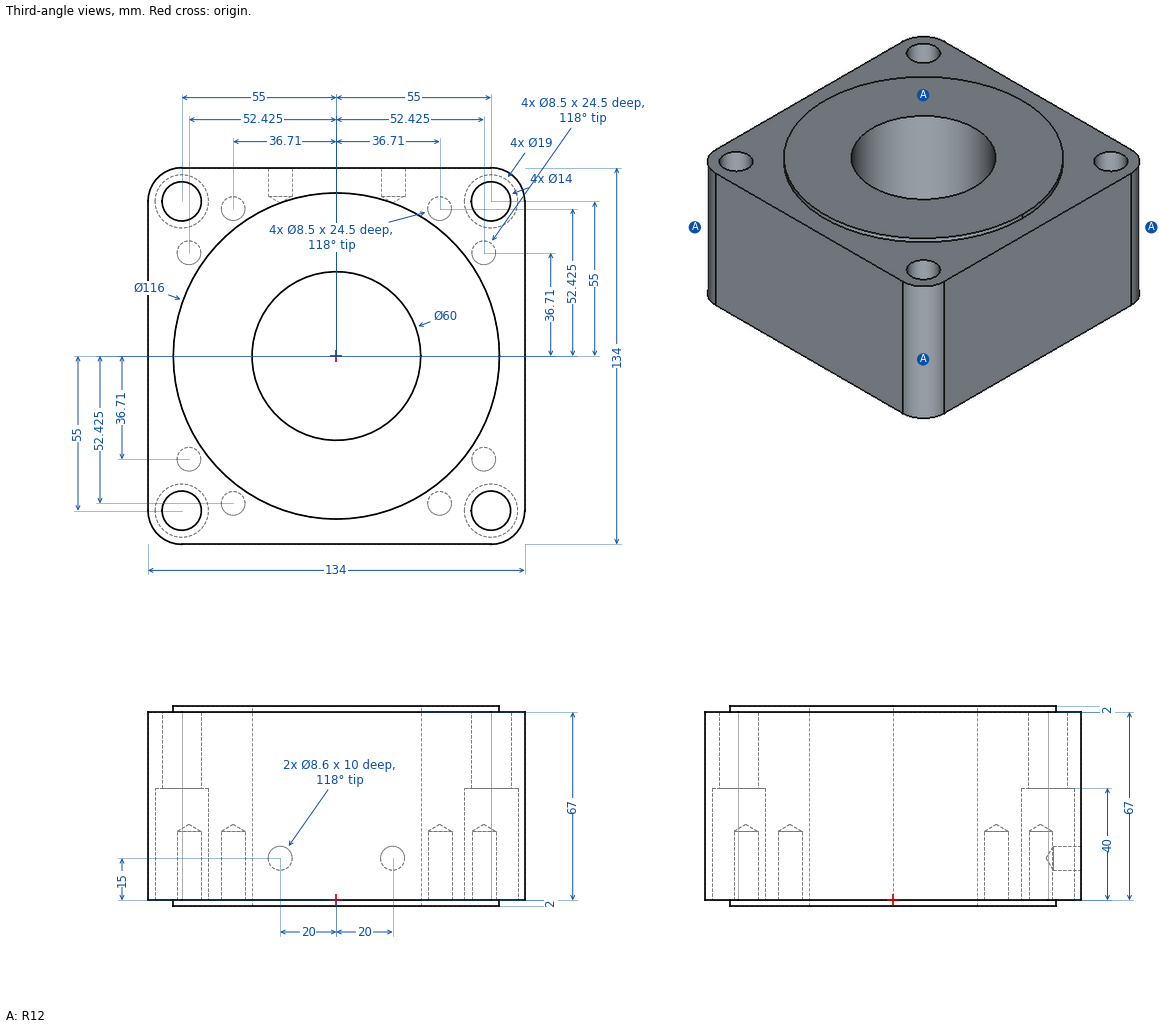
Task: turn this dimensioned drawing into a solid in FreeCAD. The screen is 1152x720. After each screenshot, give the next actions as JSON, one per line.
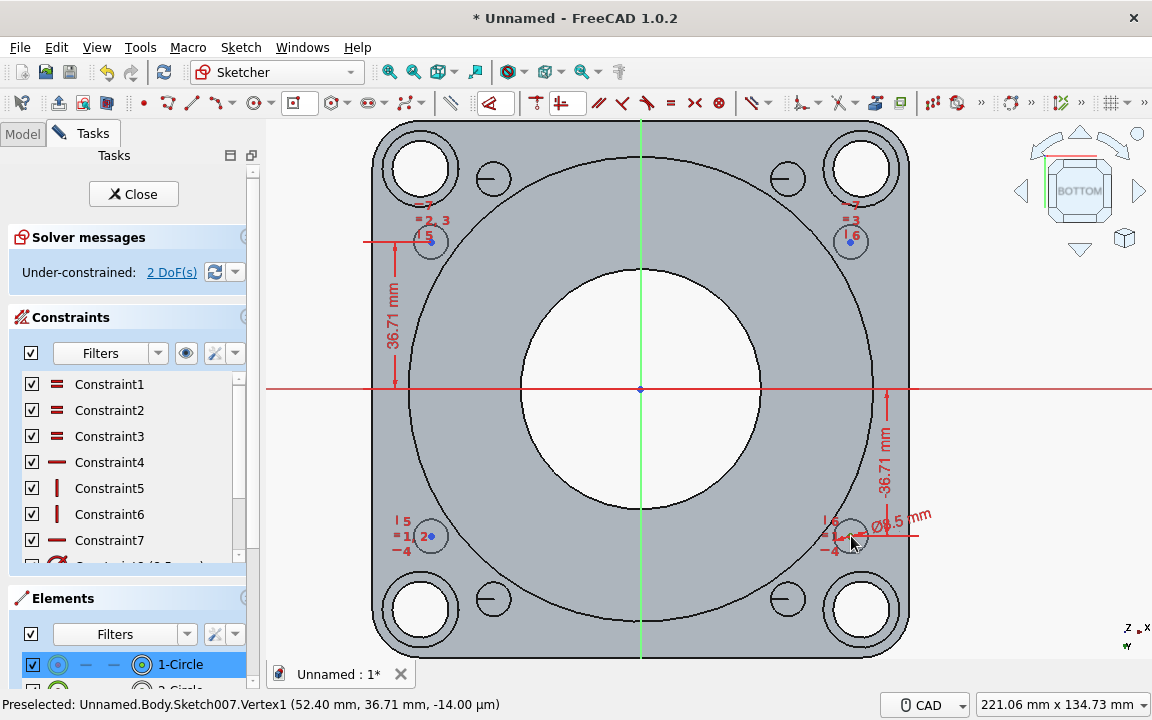
{"action": "left_click", "coordinate": [508, 104]}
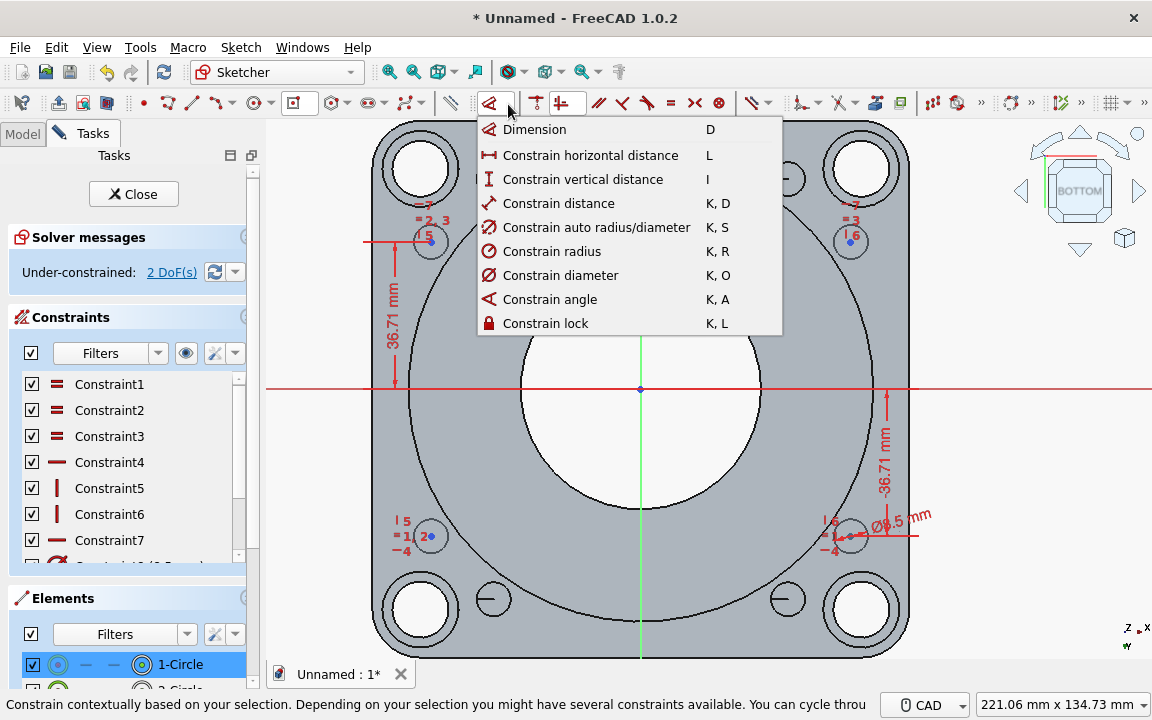
{"action": "left_click", "coordinate": [630, 155]}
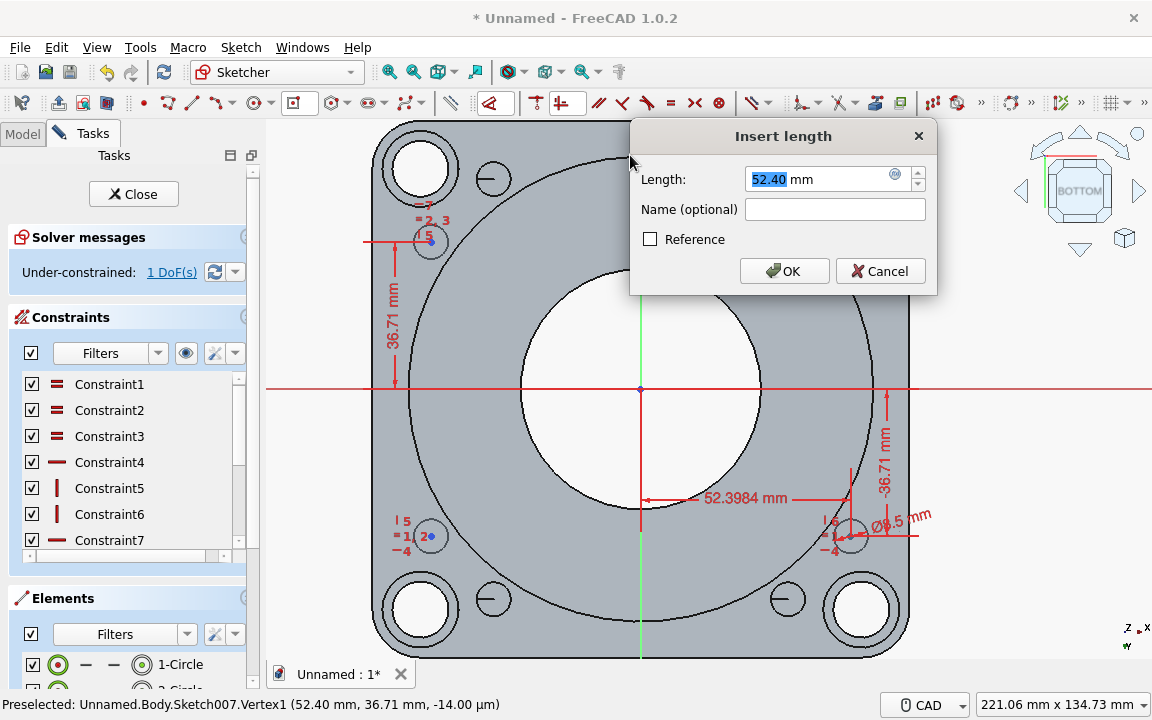
{"action": "type", "text": "52.425"}
{"action": "key", "text": "Return"}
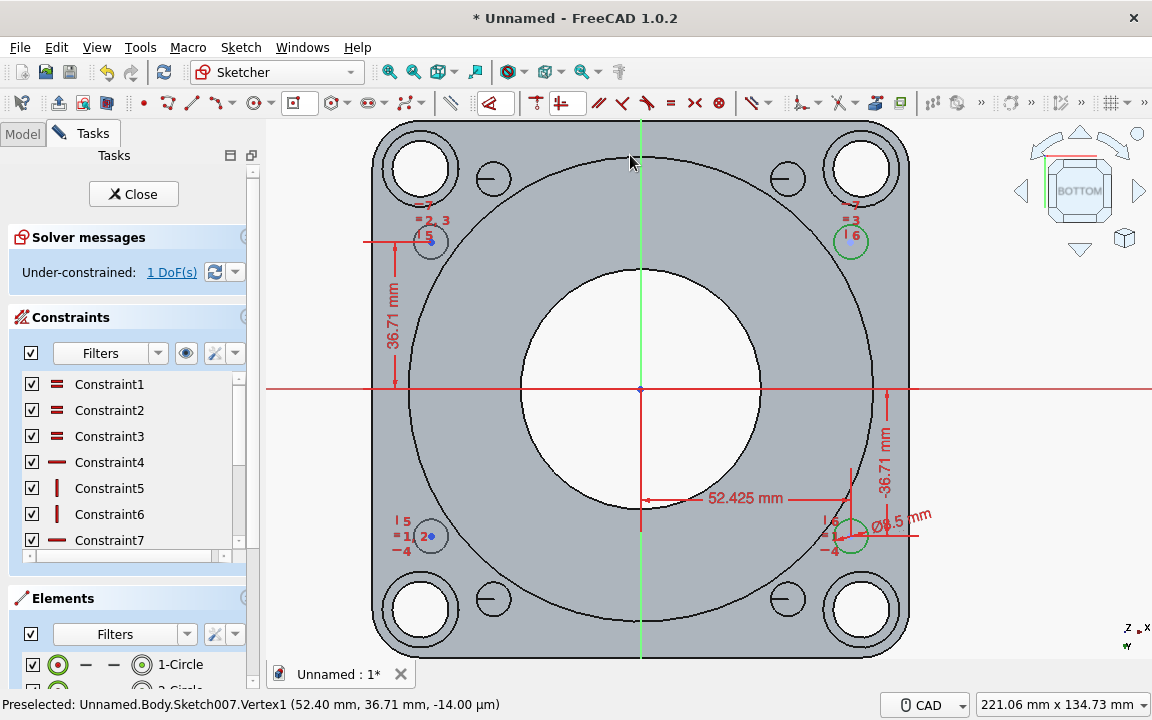
{"action": "left_click", "coordinate": [431, 536]}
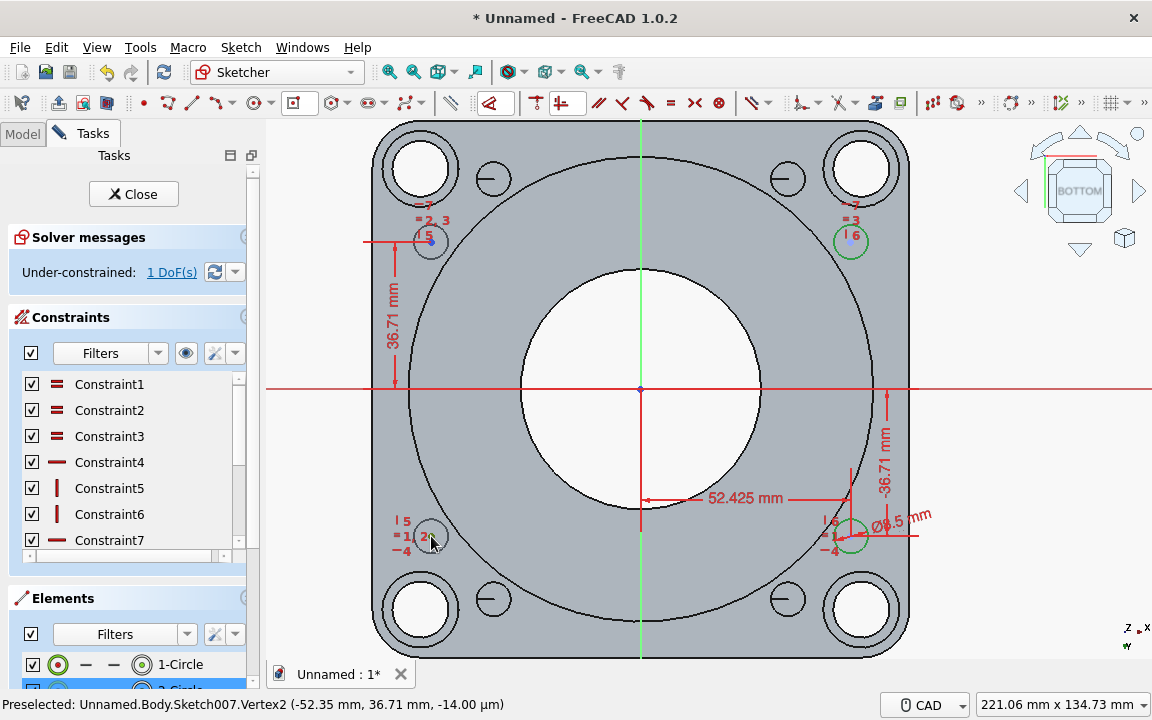
{"action": "left_click", "coordinate": [508, 104]}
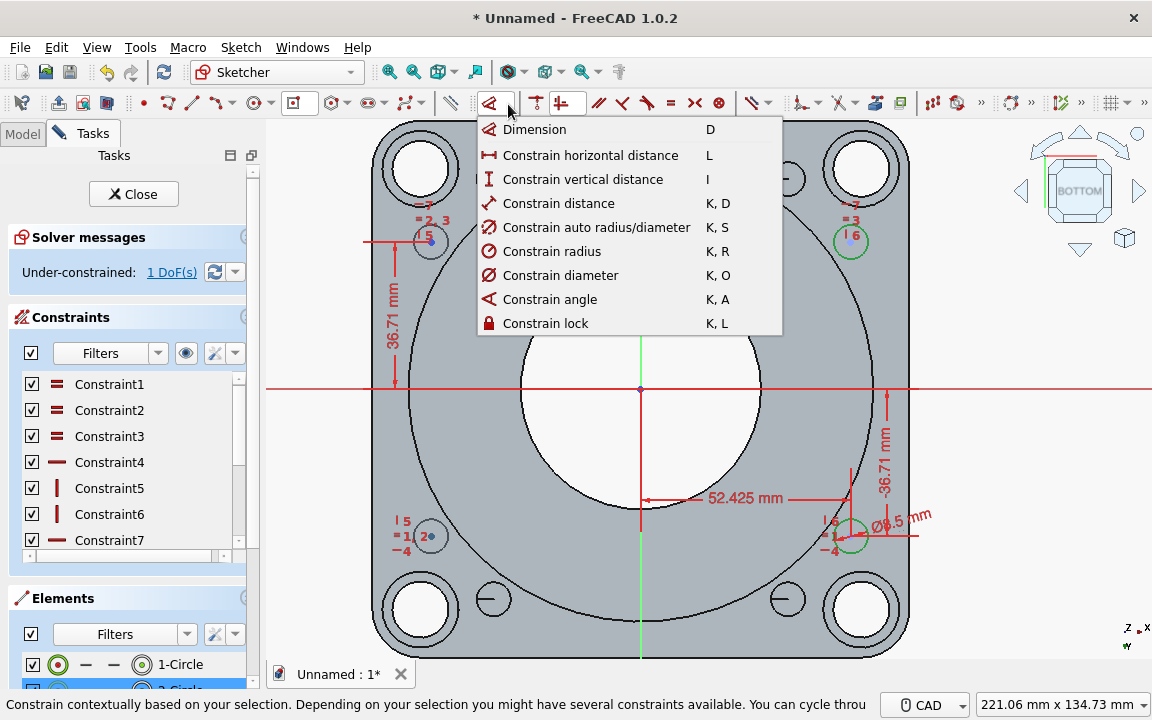
{"action": "left_click", "coordinate": [630, 155]}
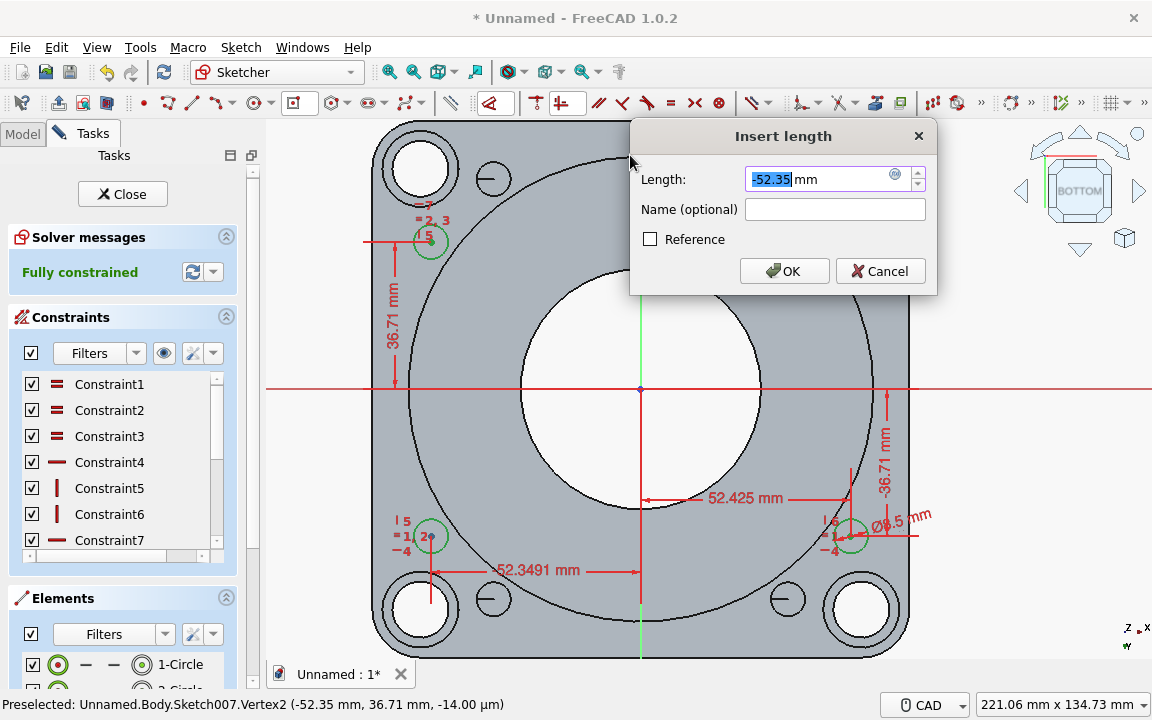
{"action": "type", "text": "-52.425"}
{"action": "key", "text": "Return"}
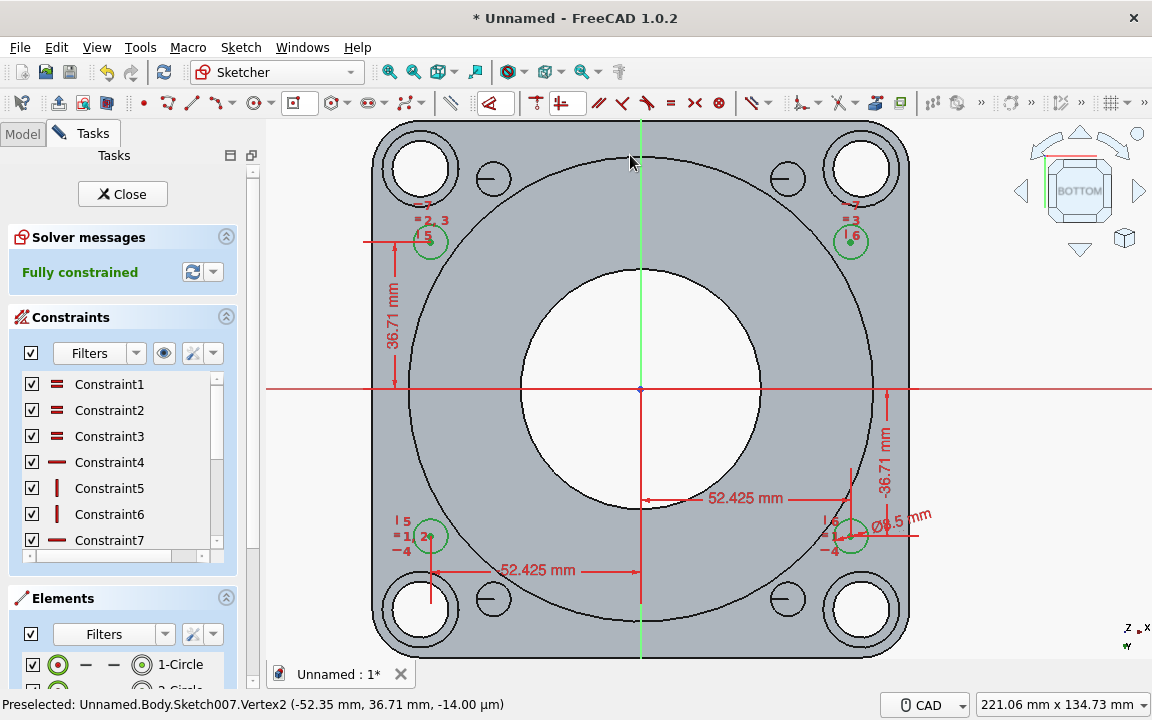
{"action": "left_click", "coordinate": [123, 194]}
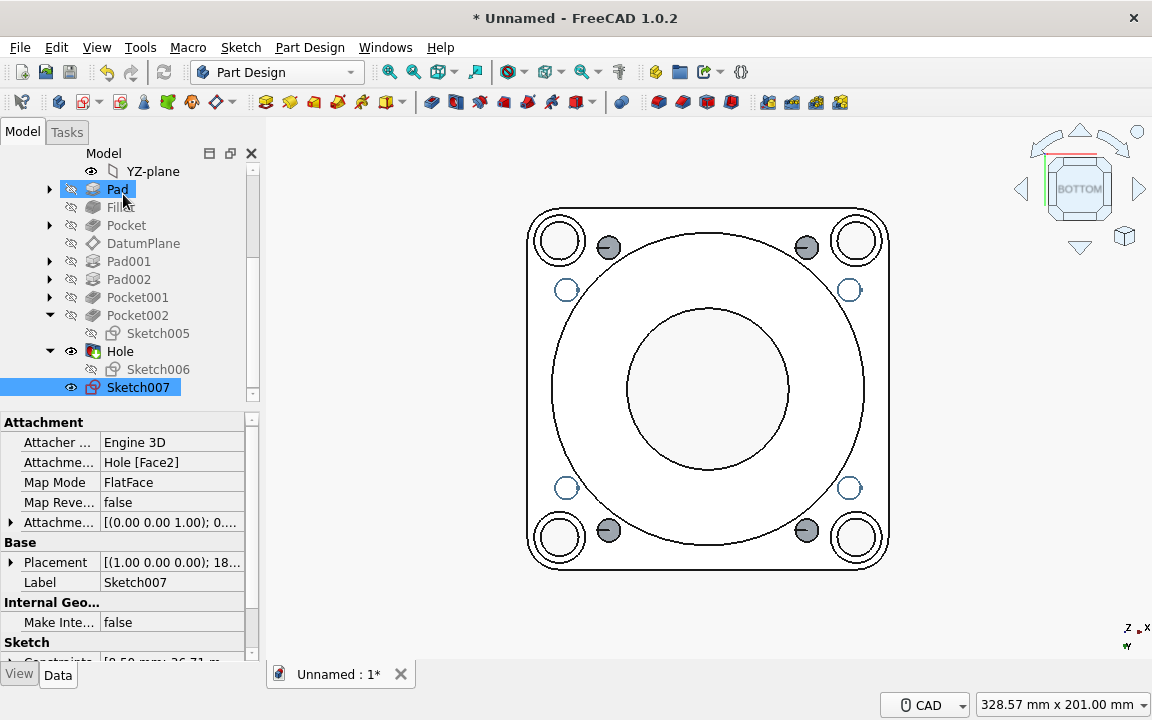
{"action": "left_click", "coordinate": [456, 102]}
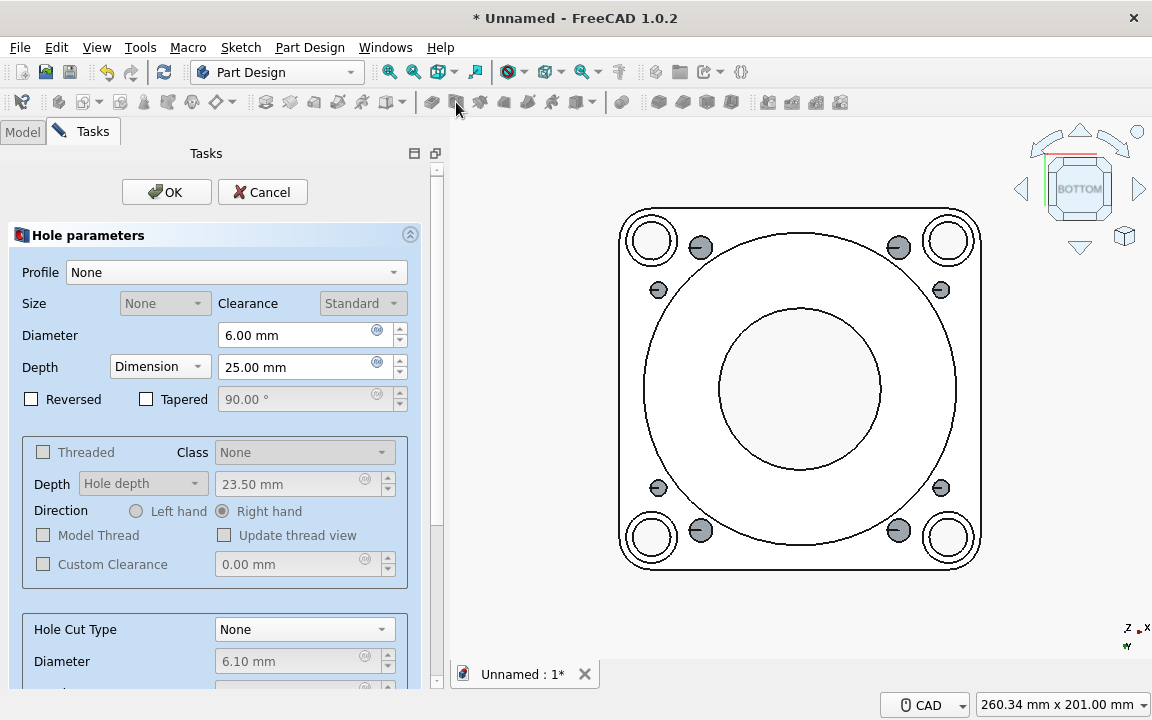
{"action": "triple_click", "coordinate": [305, 335]}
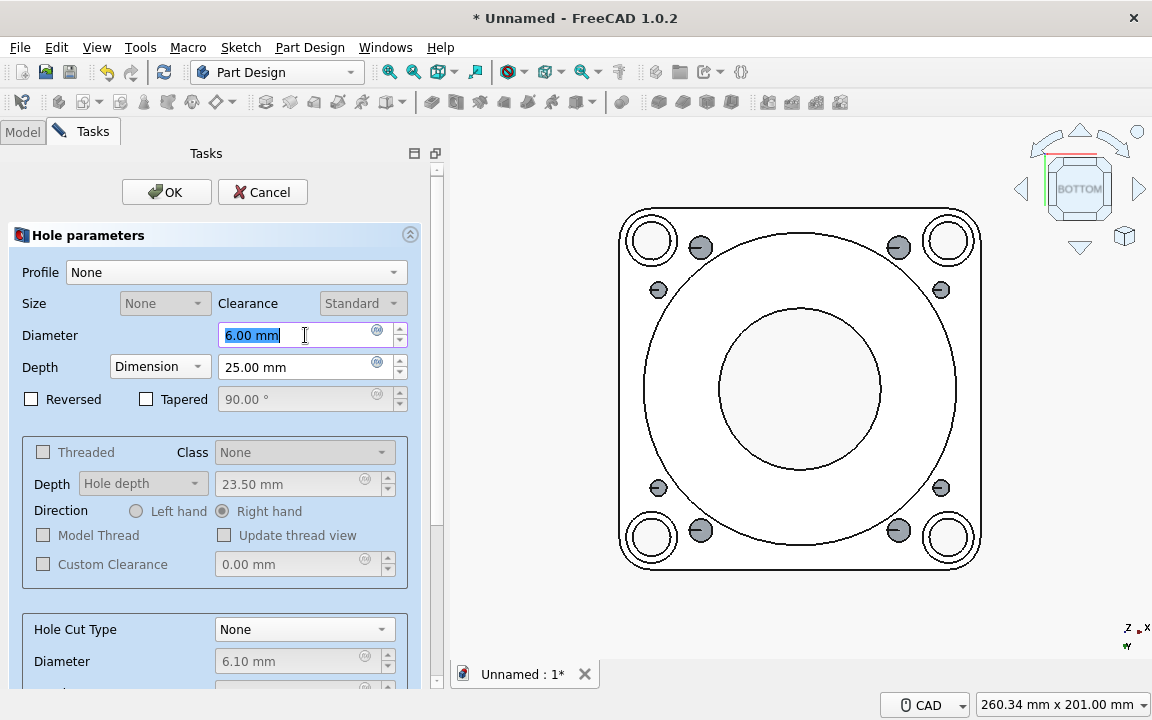
{"action": "type", "text": "8.5"}
{"action": "key", "text": "Tab"}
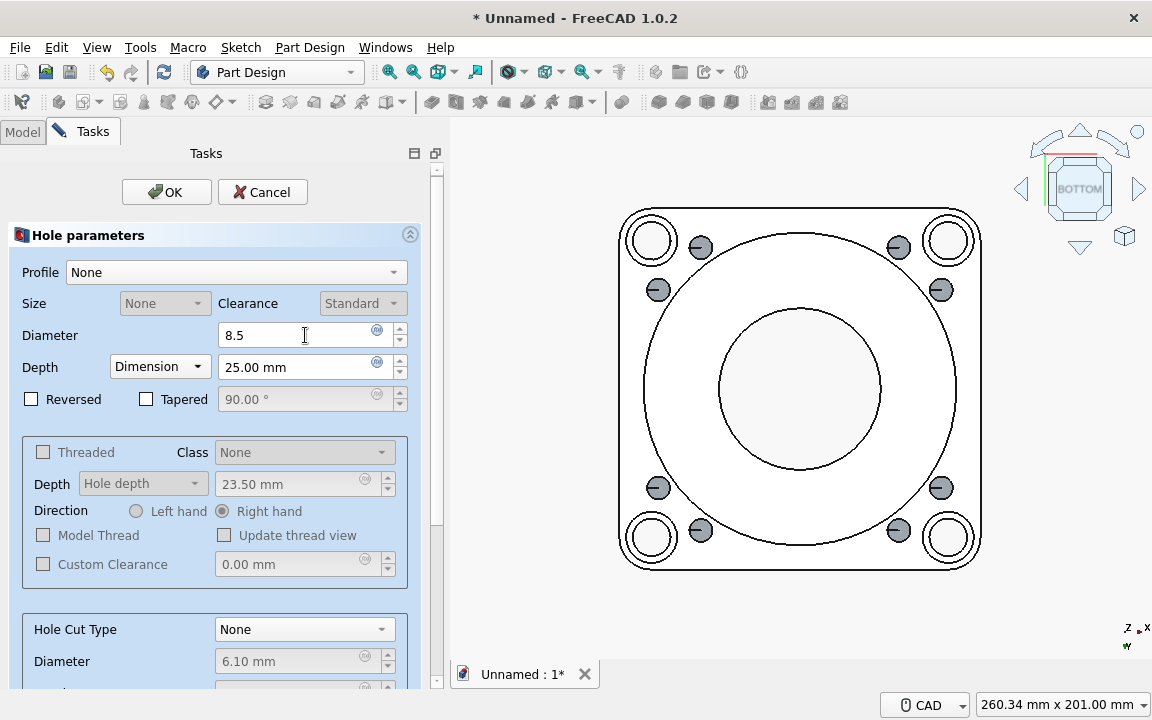
{"action": "triple_click", "coordinate": [305, 367]}